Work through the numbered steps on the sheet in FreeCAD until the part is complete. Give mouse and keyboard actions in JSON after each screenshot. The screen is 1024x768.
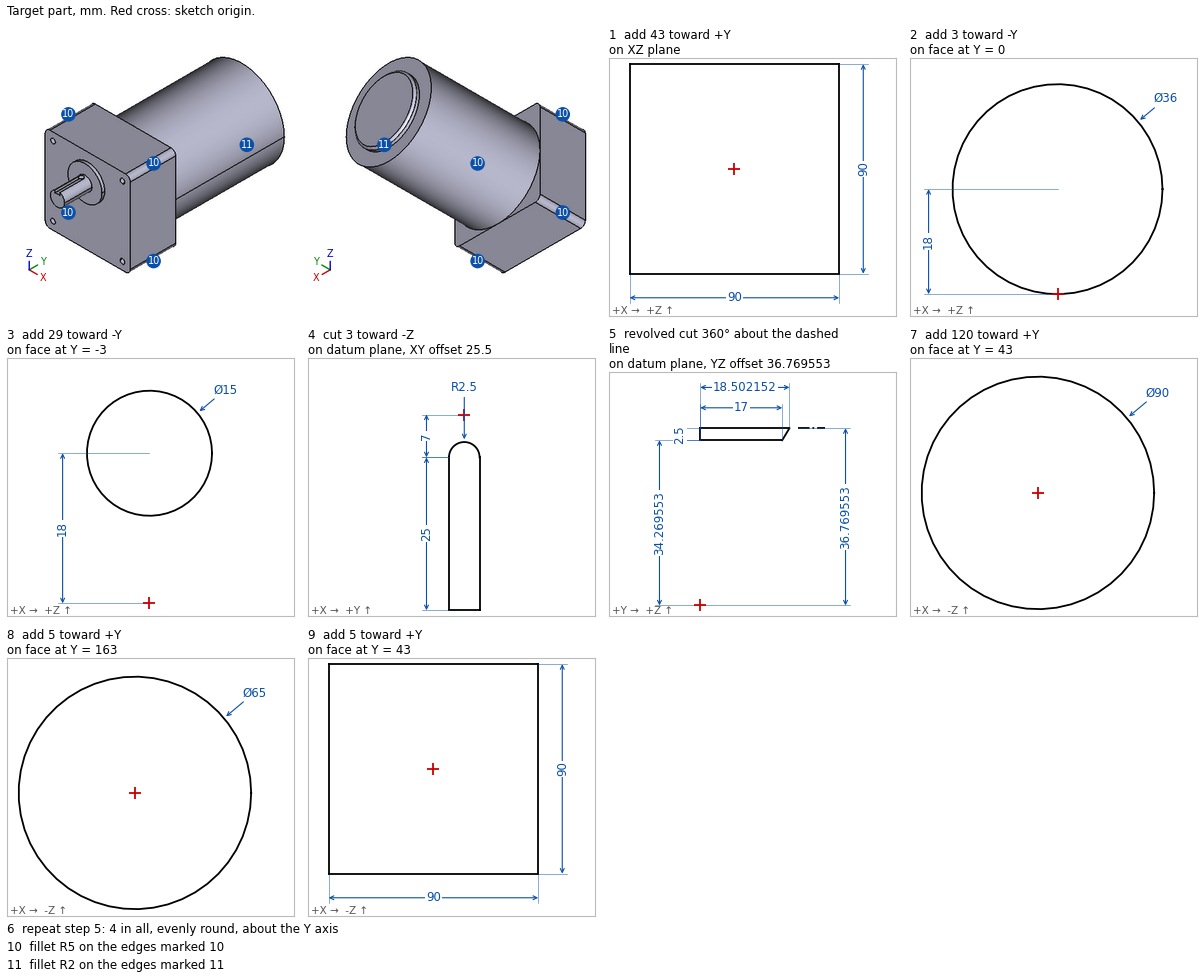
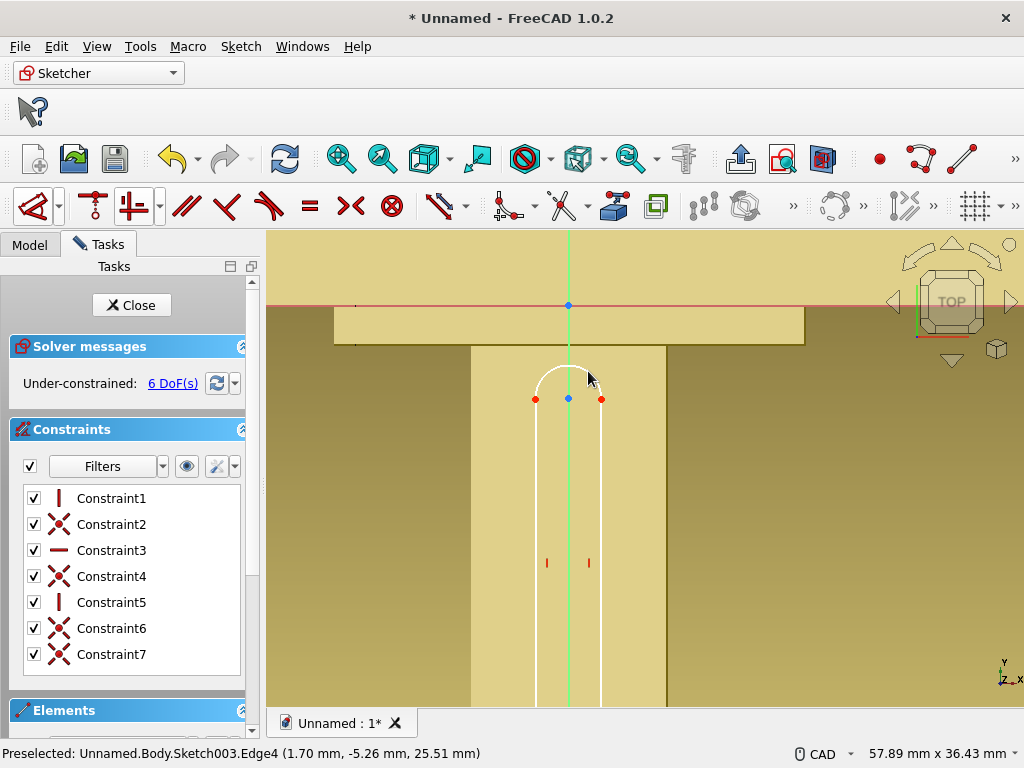
{"action": "left_click", "coordinate": [536, 497]}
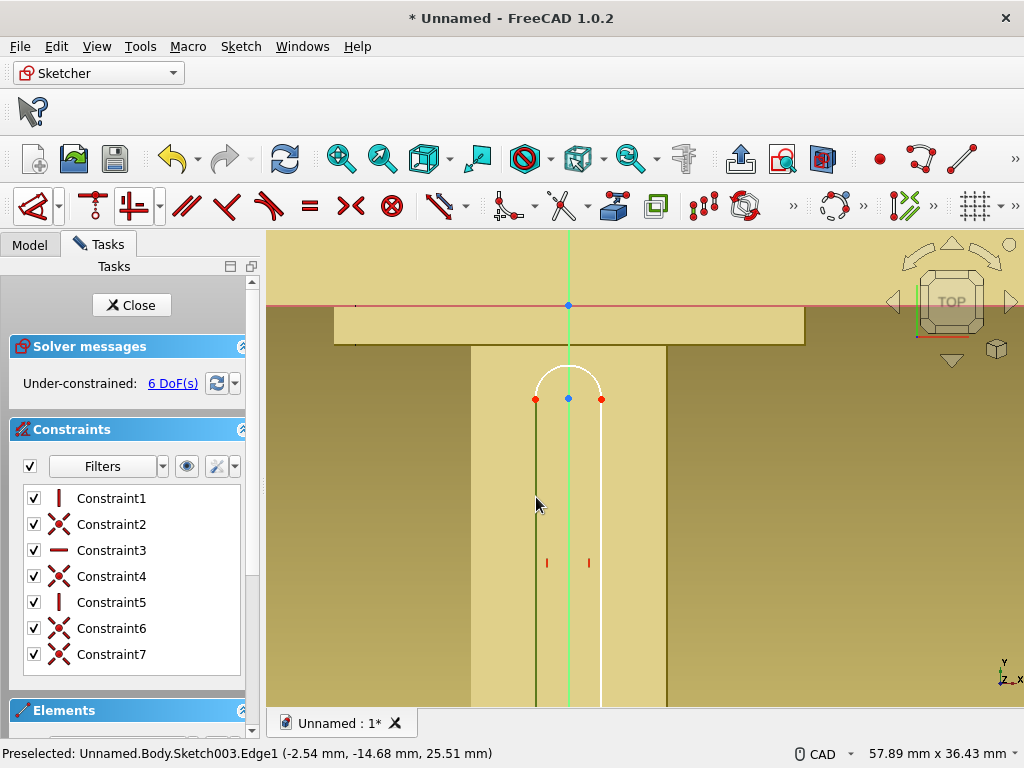
{"action": "left_click", "coordinate": [588, 372]}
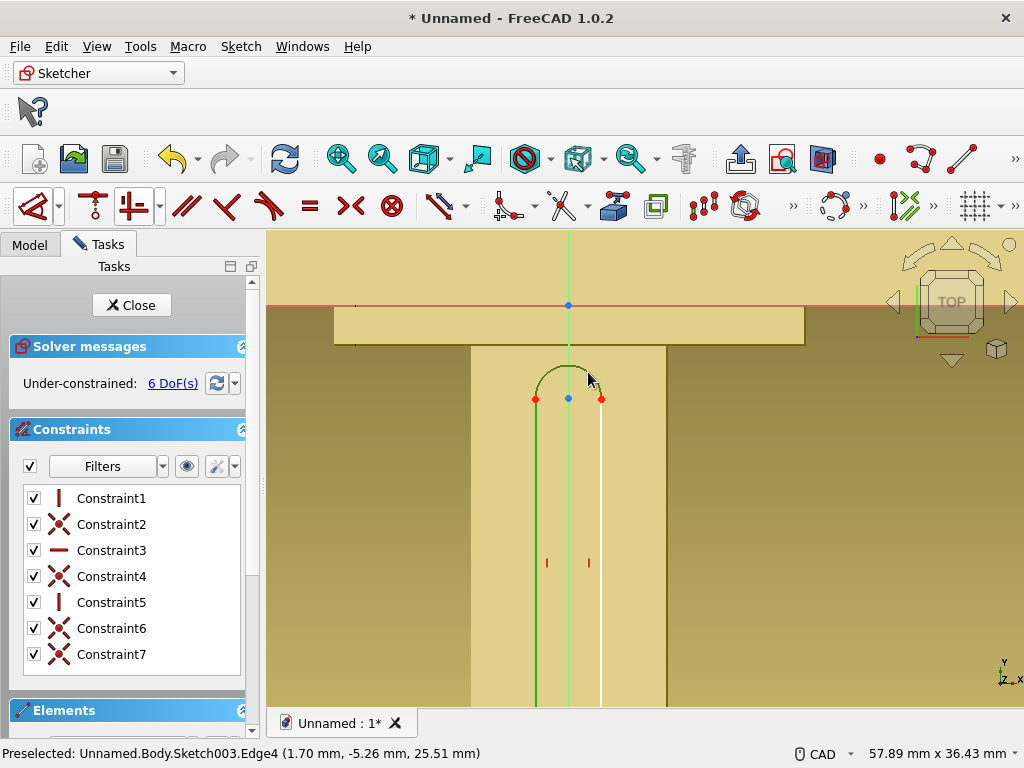
{"action": "left_click", "coordinate": [269, 206]}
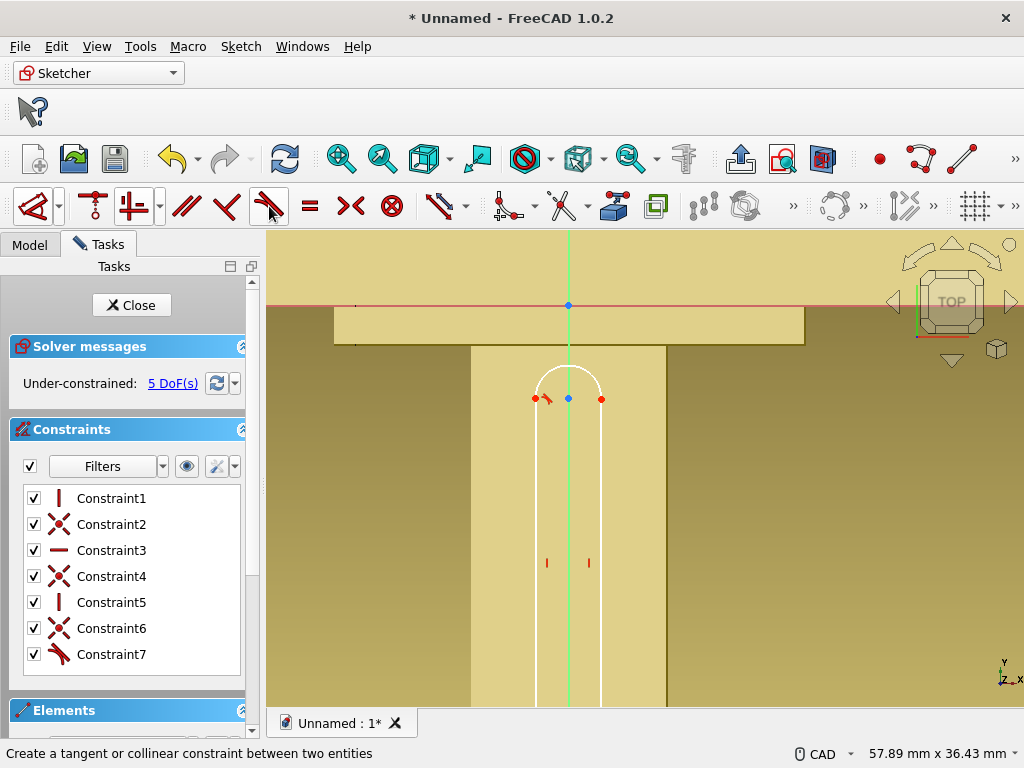
{"action": "left_click", "coordinate": [601, 628]}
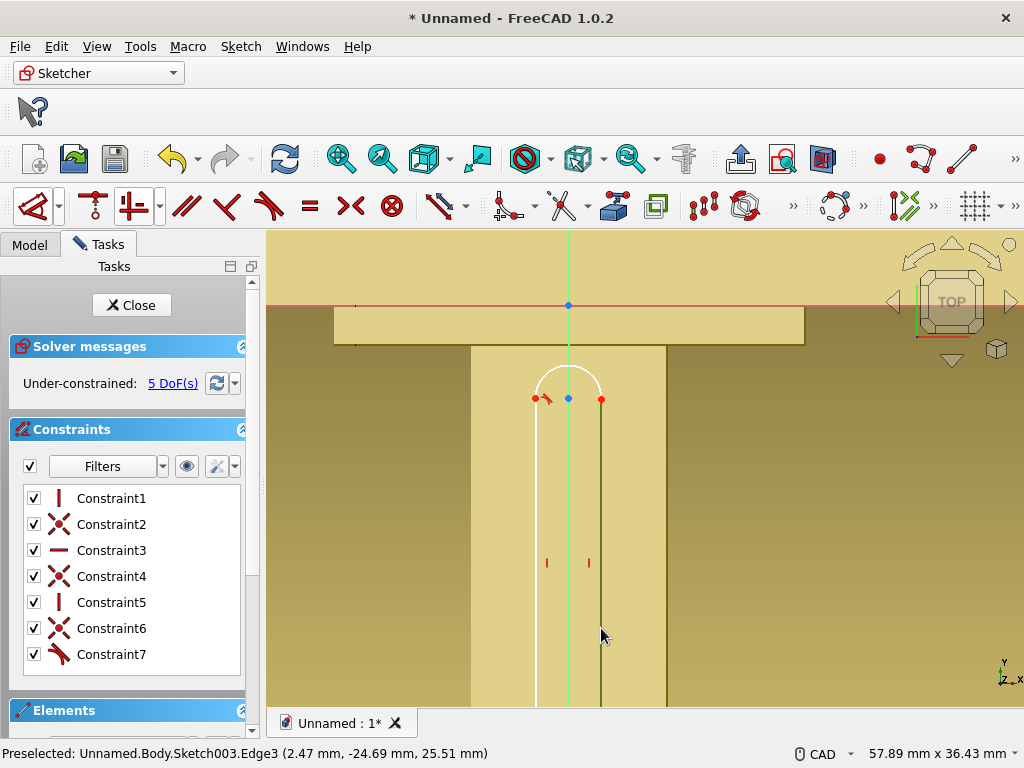
{"action": "left_click", "coordinate": [588, 372]}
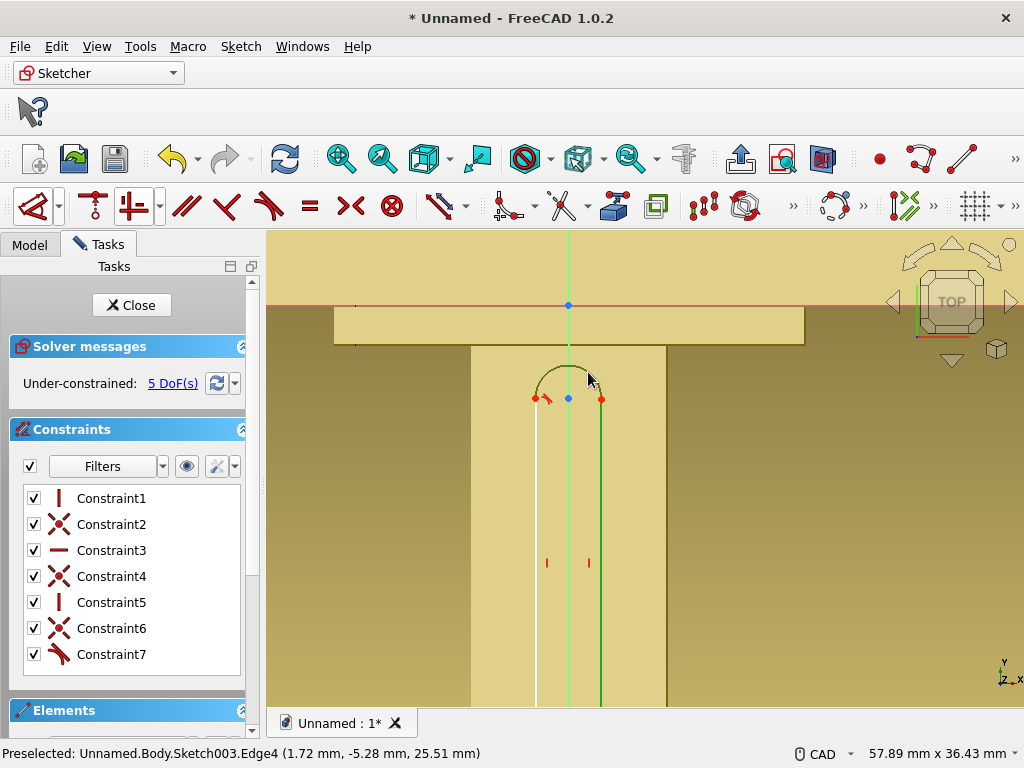
{"action": "left_click", "coordinate": [269, 206]}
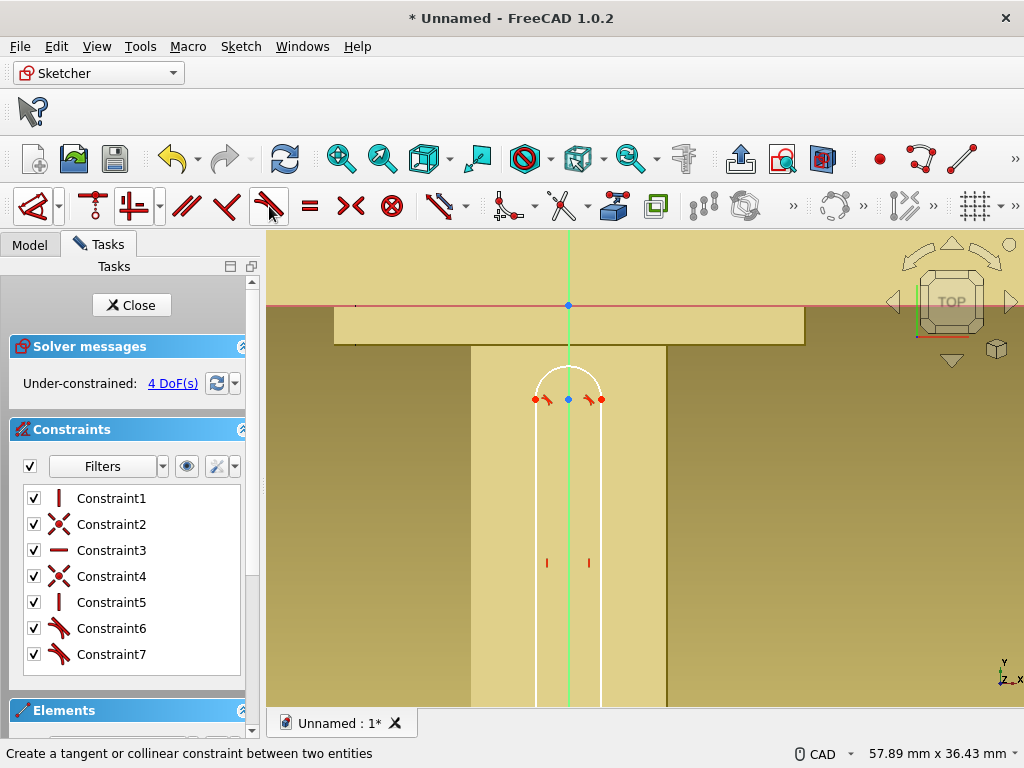
{"action": "left_click", "coordinate": [568, 399]}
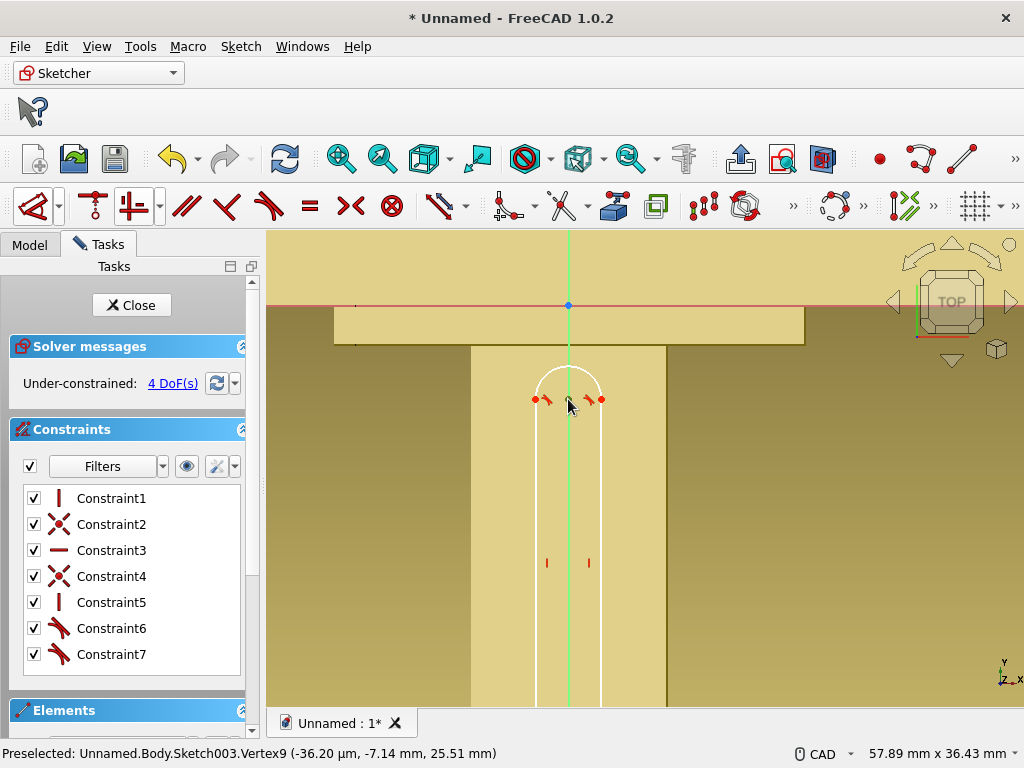
{"action": "left_click", "coordinate": [569, 649]}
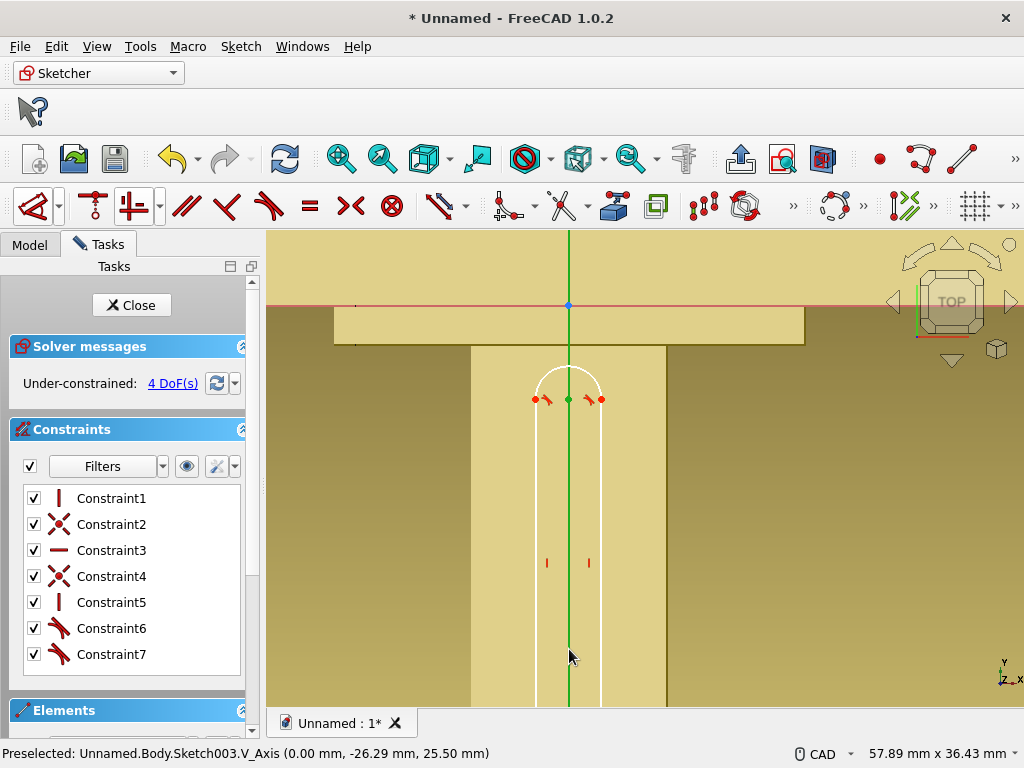
{"action": "left_click", "coordinate": [93, 206]}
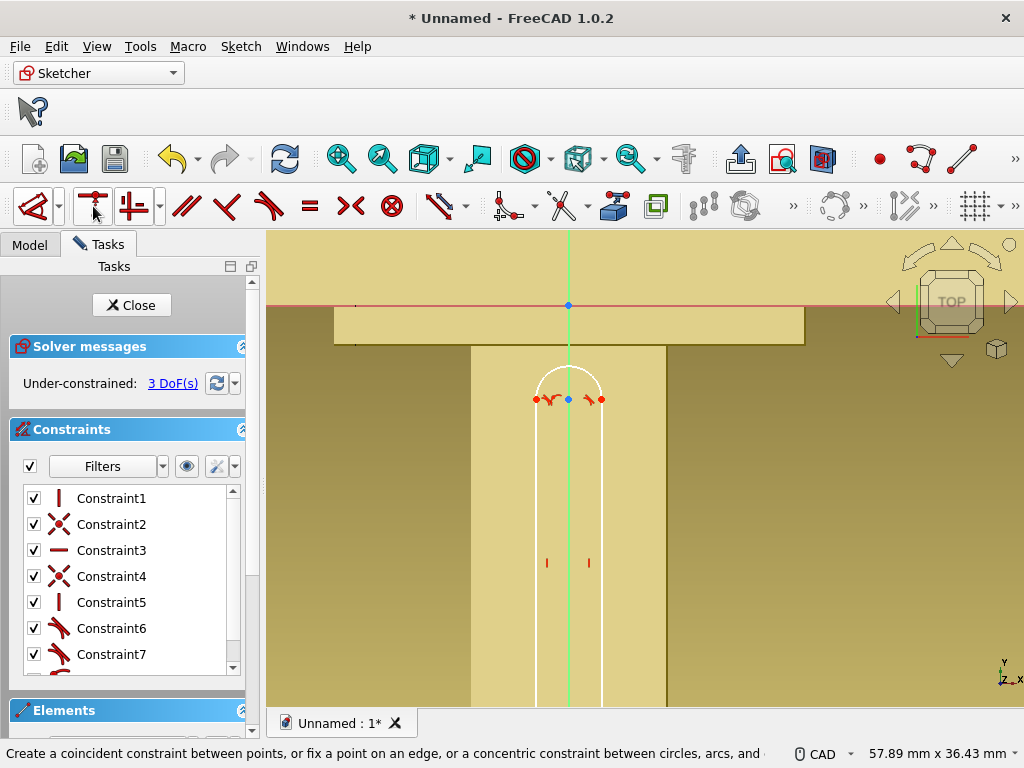
{"action": "left_click", "coordinate": [588, 373]}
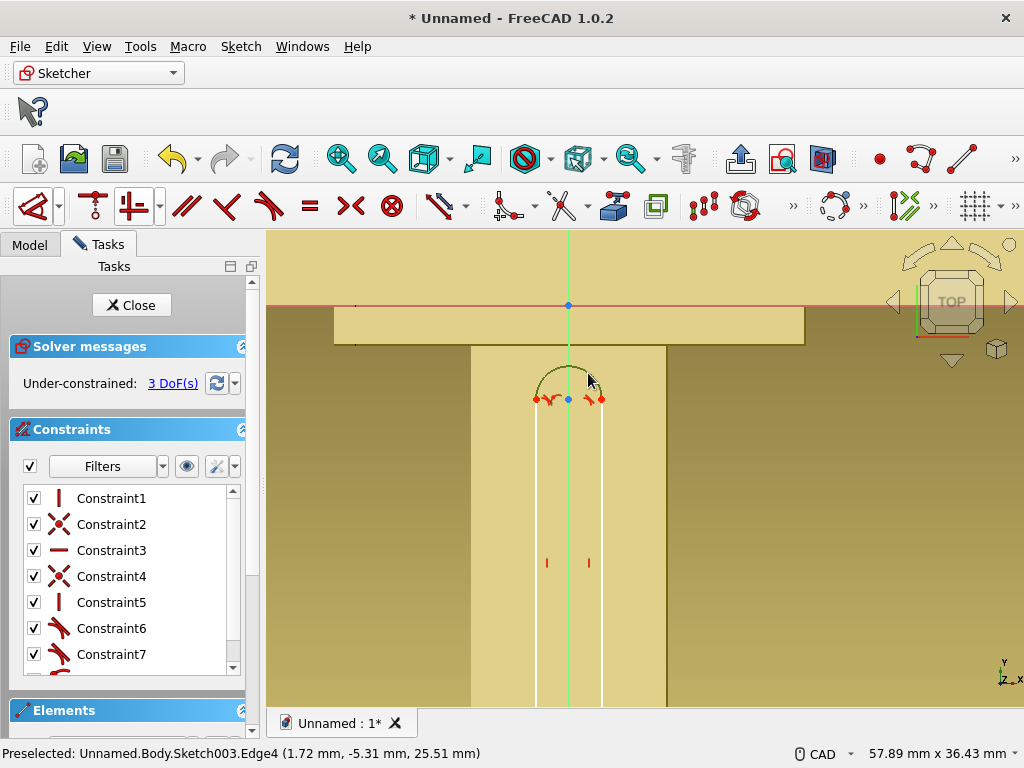
{"action": "left_click", "coordinate": [58, 206]}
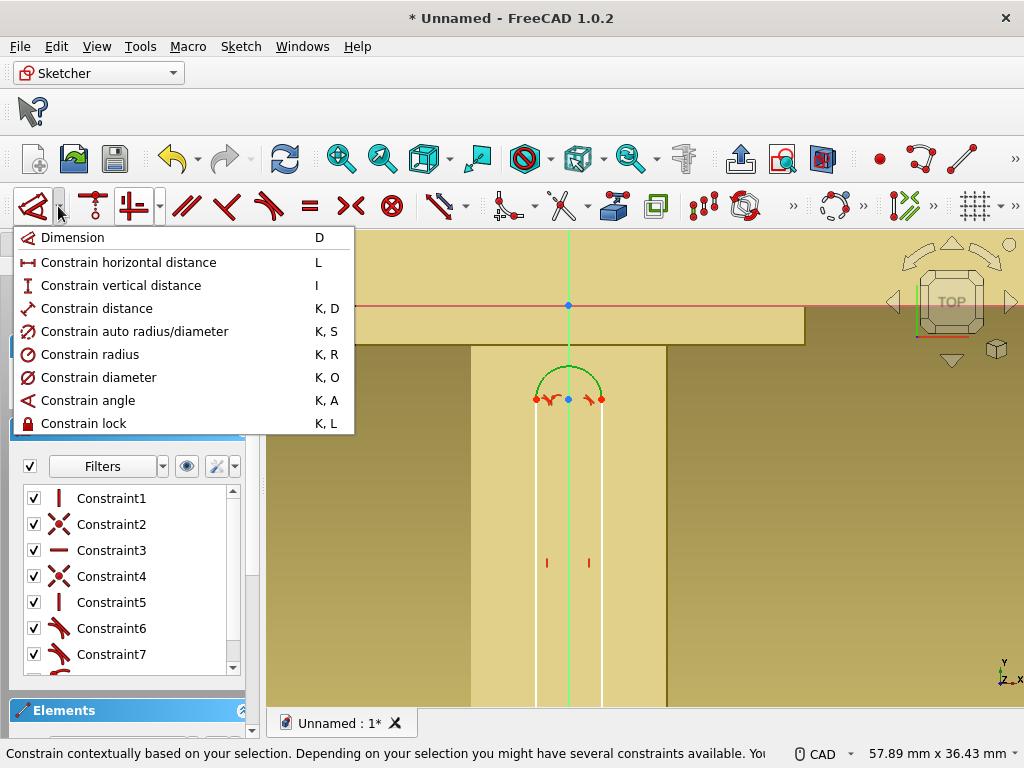
{"action": "left_click", "coordinate": [184, 354]}